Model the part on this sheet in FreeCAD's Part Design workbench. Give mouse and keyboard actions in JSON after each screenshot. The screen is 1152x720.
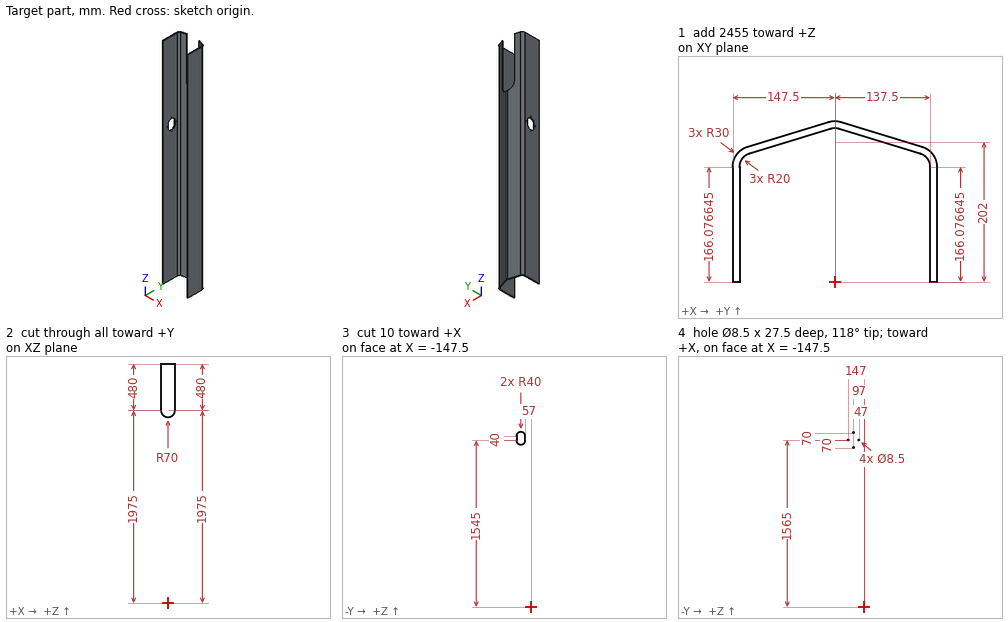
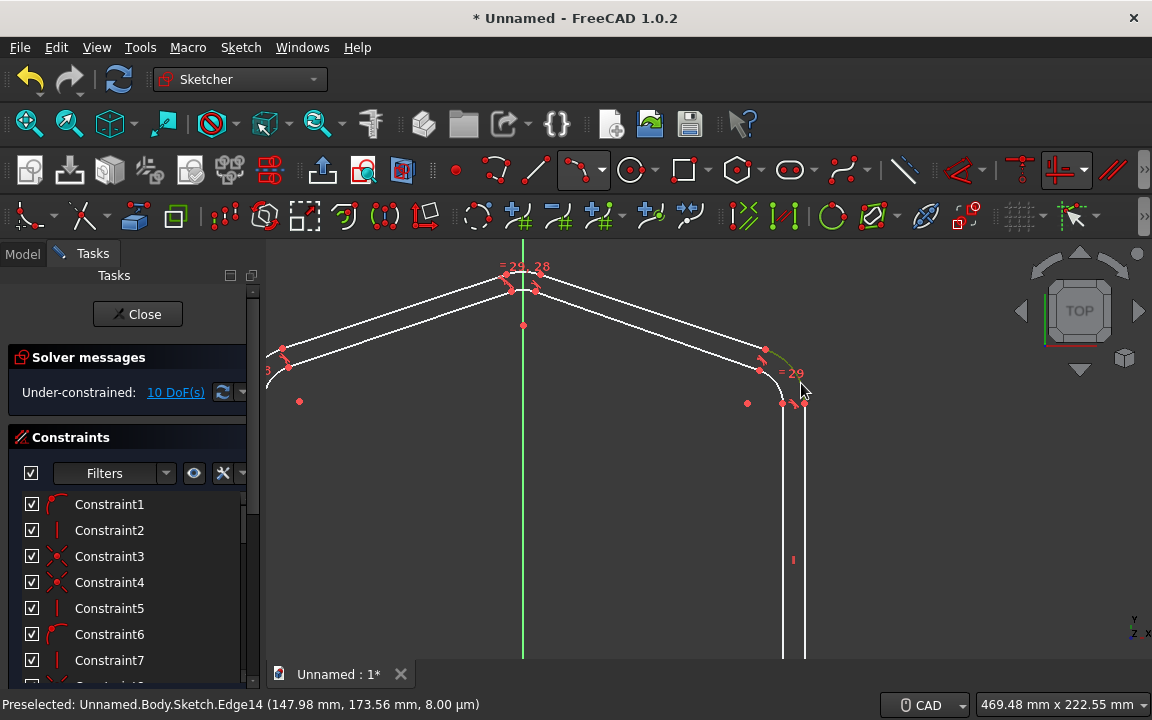
{"action": "scroll", "coordinate": [523, 272], "scroll_direction": "up", "scroll_amount": 4}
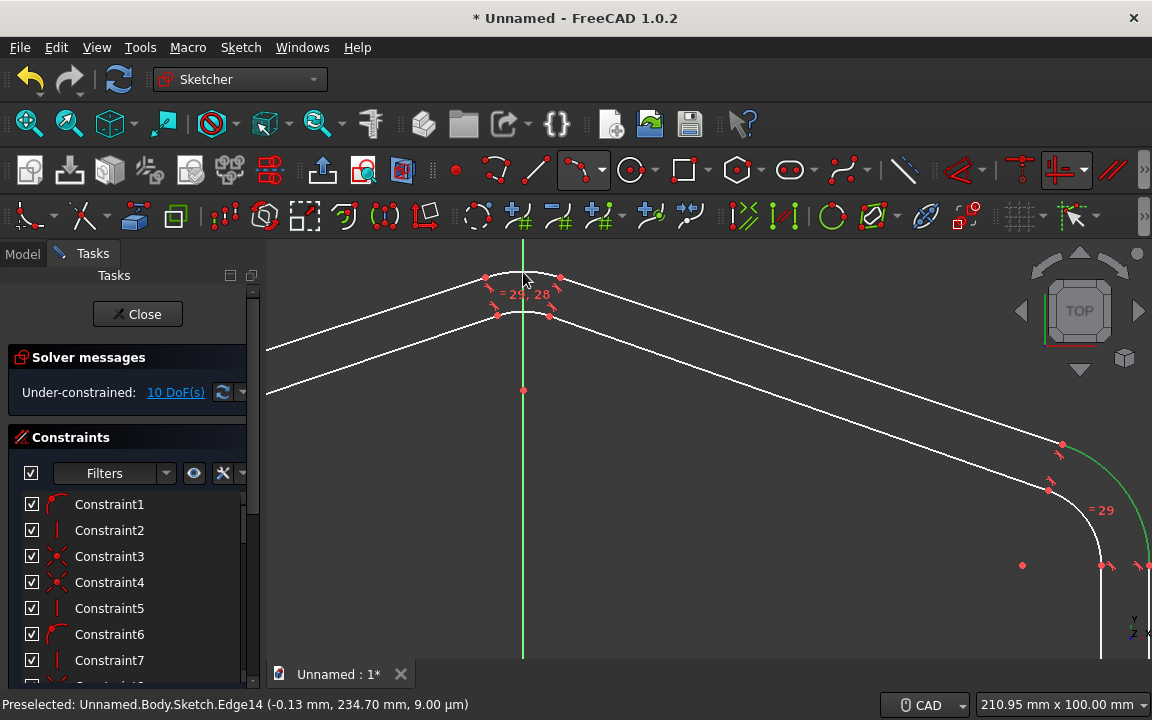
{"action": "left_click", "coordinate": [523, 272]}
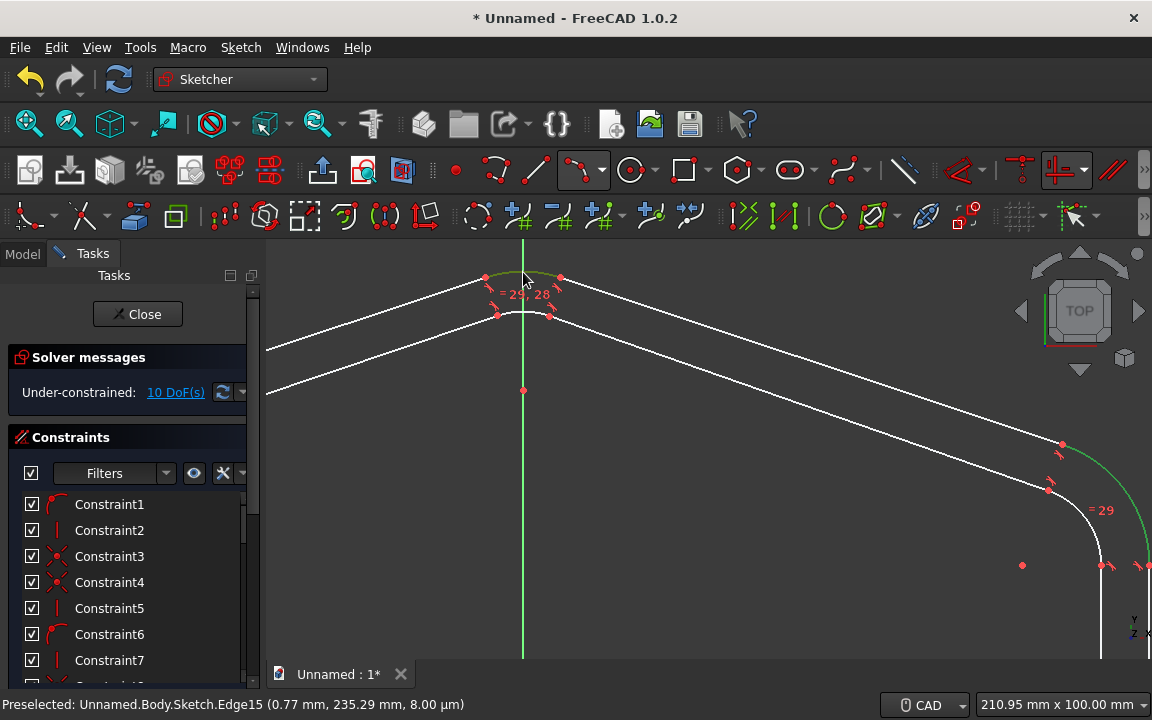
{"action": "scroll", "coordinate": [679, 343], "scroll_direction": "down", "scroll_amount": 7}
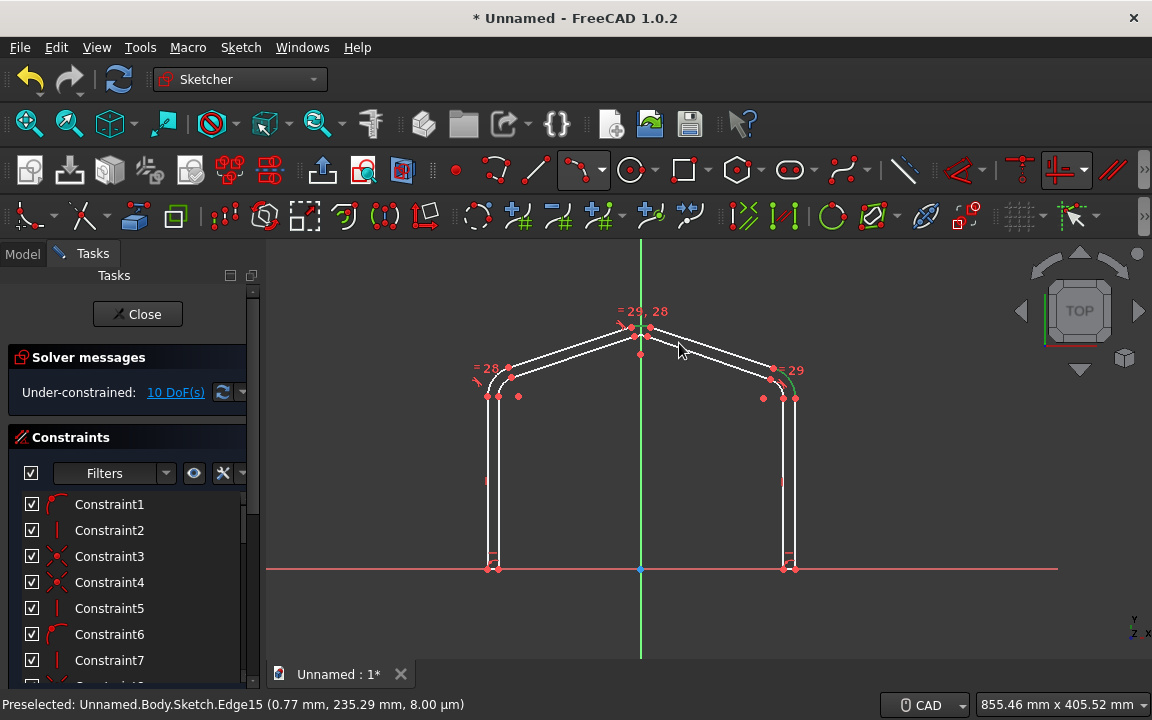
{"action": "scroll", "coordinate": [499, 373], "scroll_direction": "up", "scroll_amount": 2}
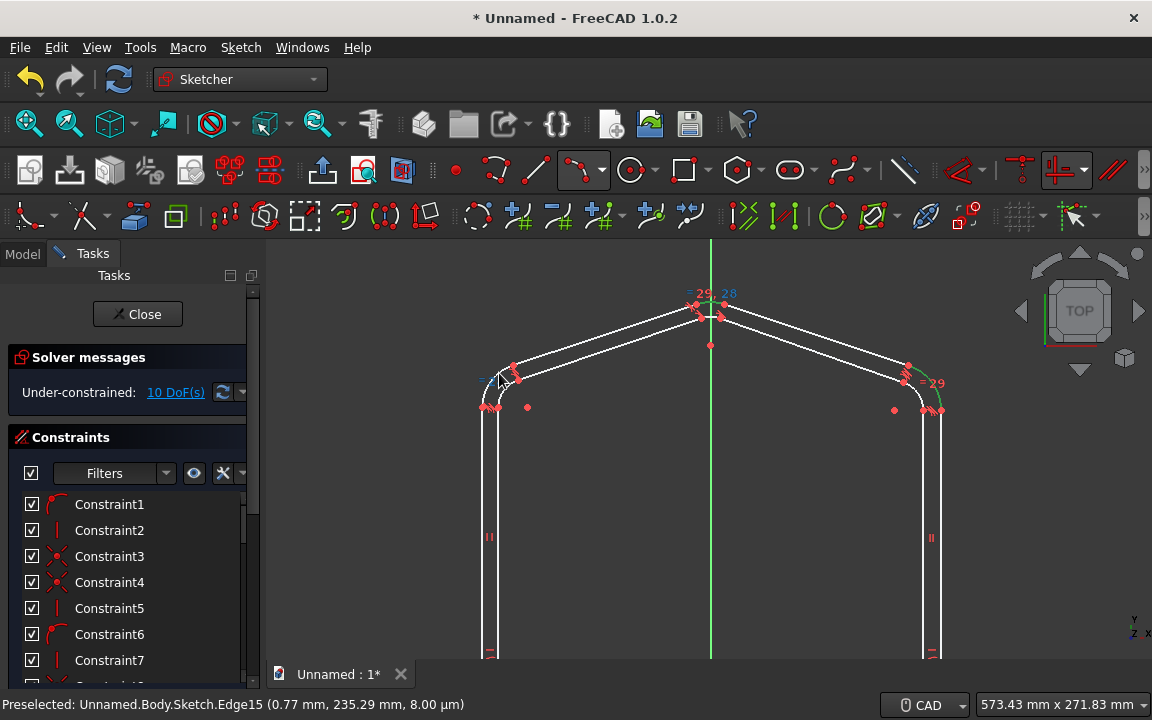
{"action": "left_click", "coordinate": [486, 391]}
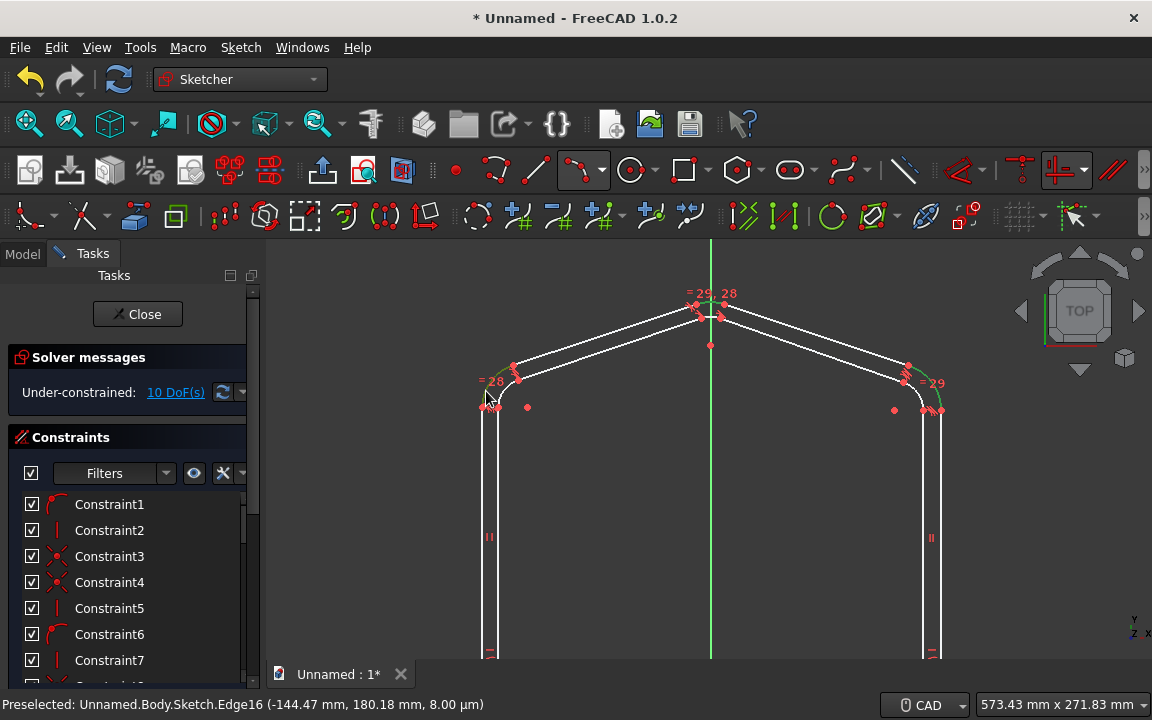
{"action": "key", "text": "e"}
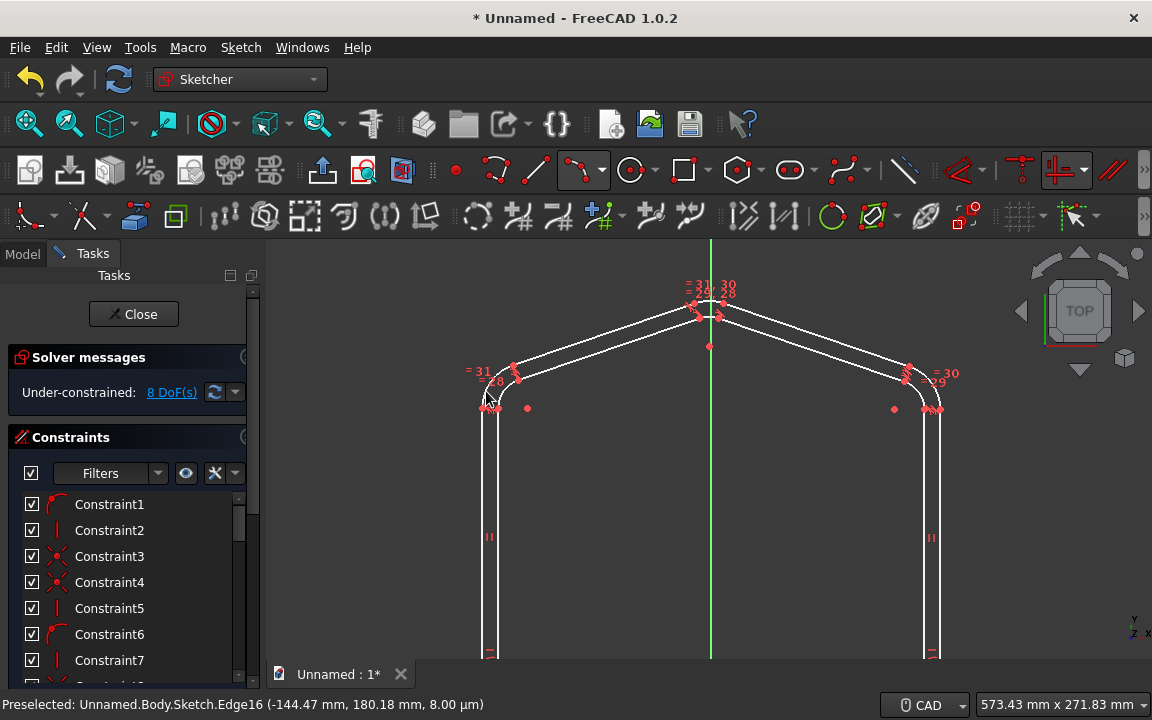
{"action": "left_click", "coordinate": [709, 346]}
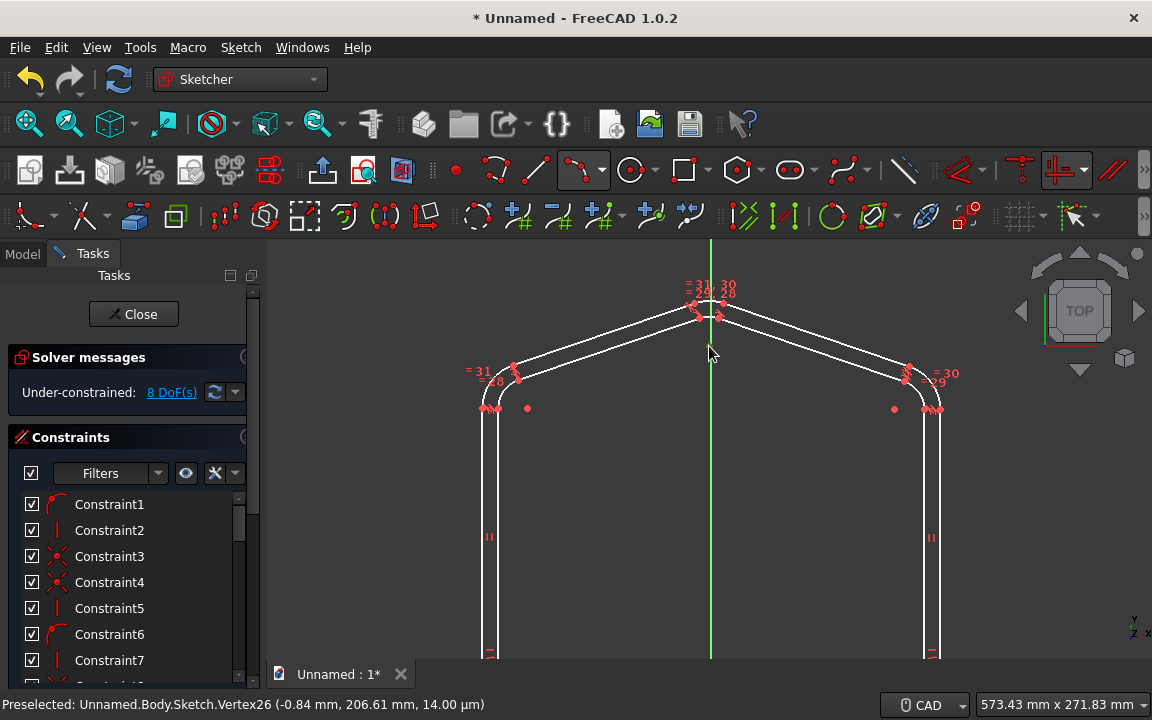
{"action": "left_click", "coordinate": [711, 605]}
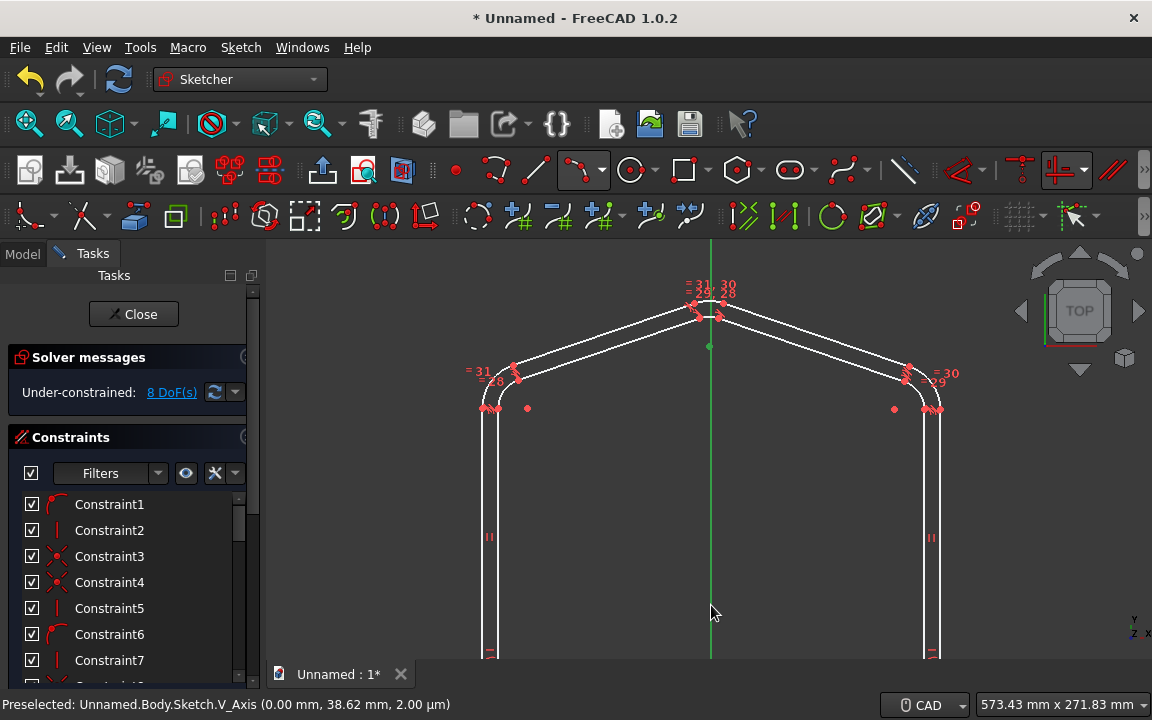
{"action": "left_click", "coordinate": [1020, 170]}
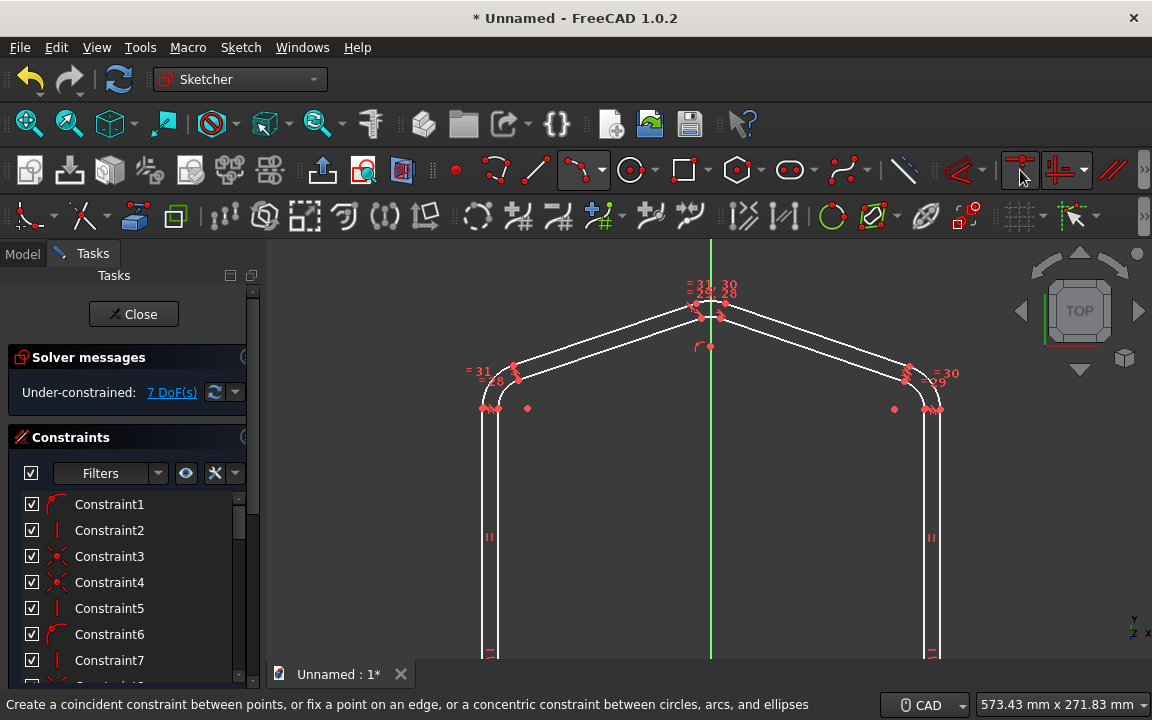
{"action": "left_click", "coordinate": [958, 170]}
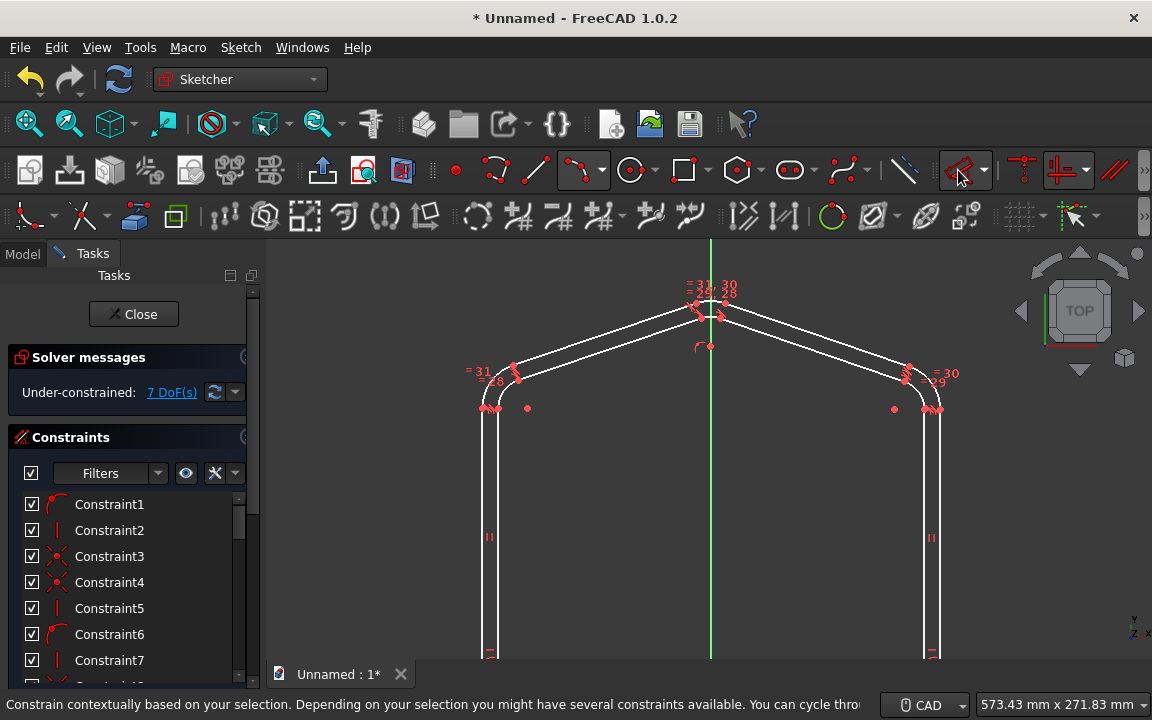
{"action": "scroll", "coordinate": [509, 386], "scroll_direction": "up", "scroll_amount": 2}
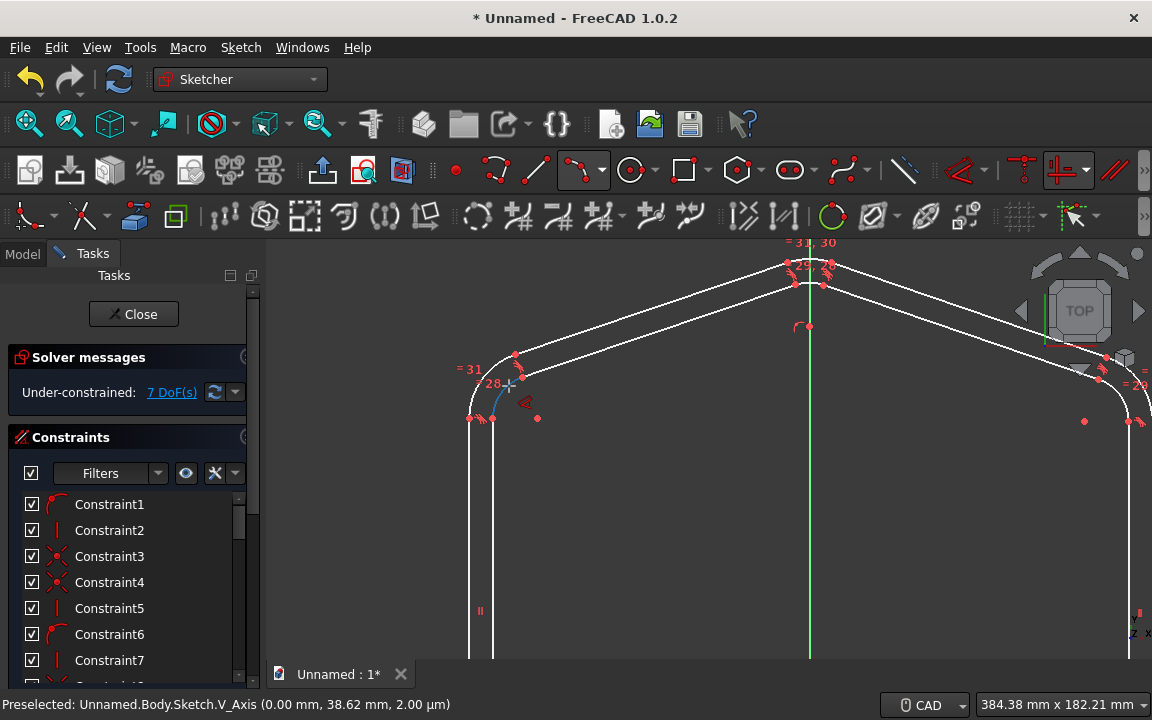
{"action": "left_click", "coordinate": [509, 385]}
{"action": "left_click", "coordinate": [596, 370]}